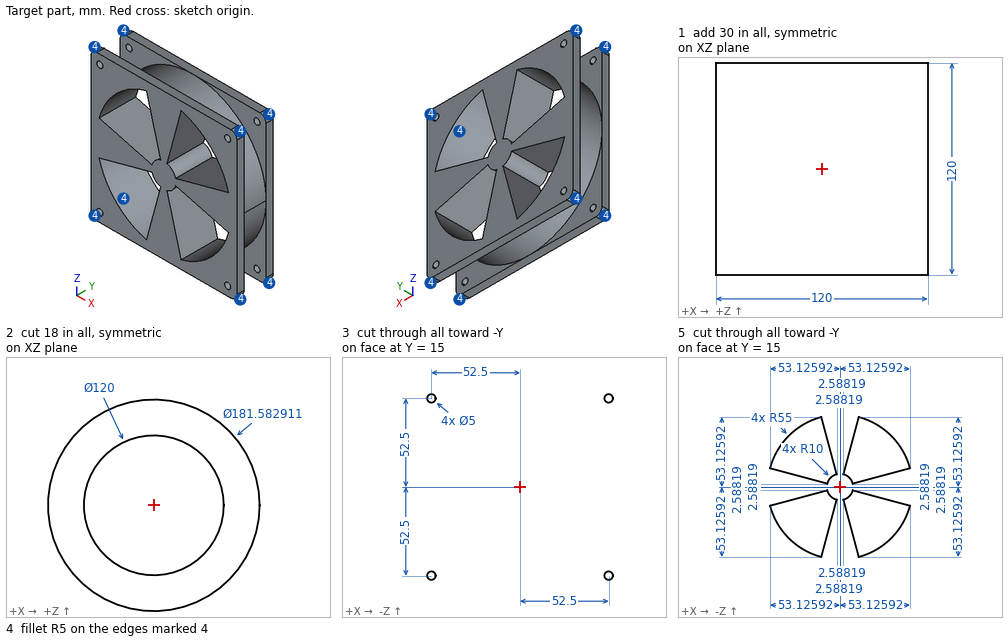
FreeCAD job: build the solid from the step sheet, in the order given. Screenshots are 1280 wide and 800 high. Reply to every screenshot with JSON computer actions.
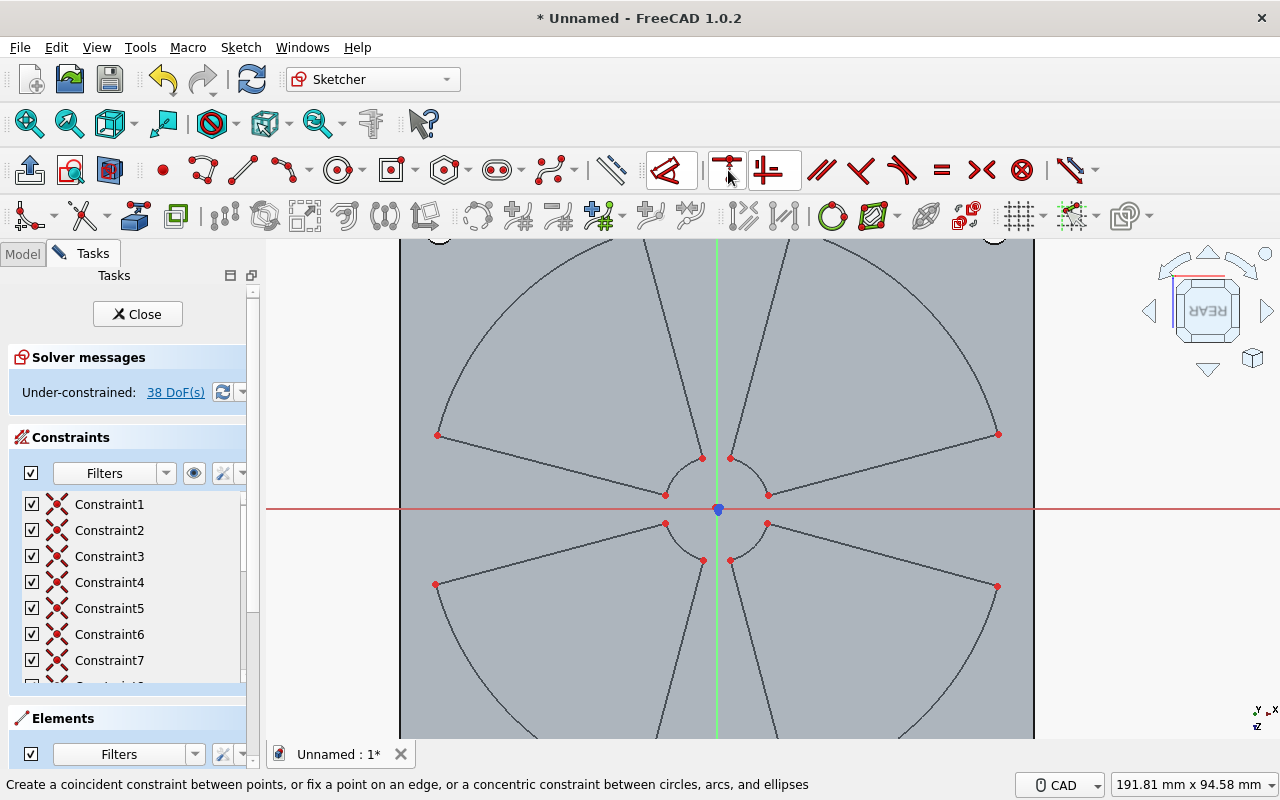
{"action": "left_click", "coordinate": [473, 353]}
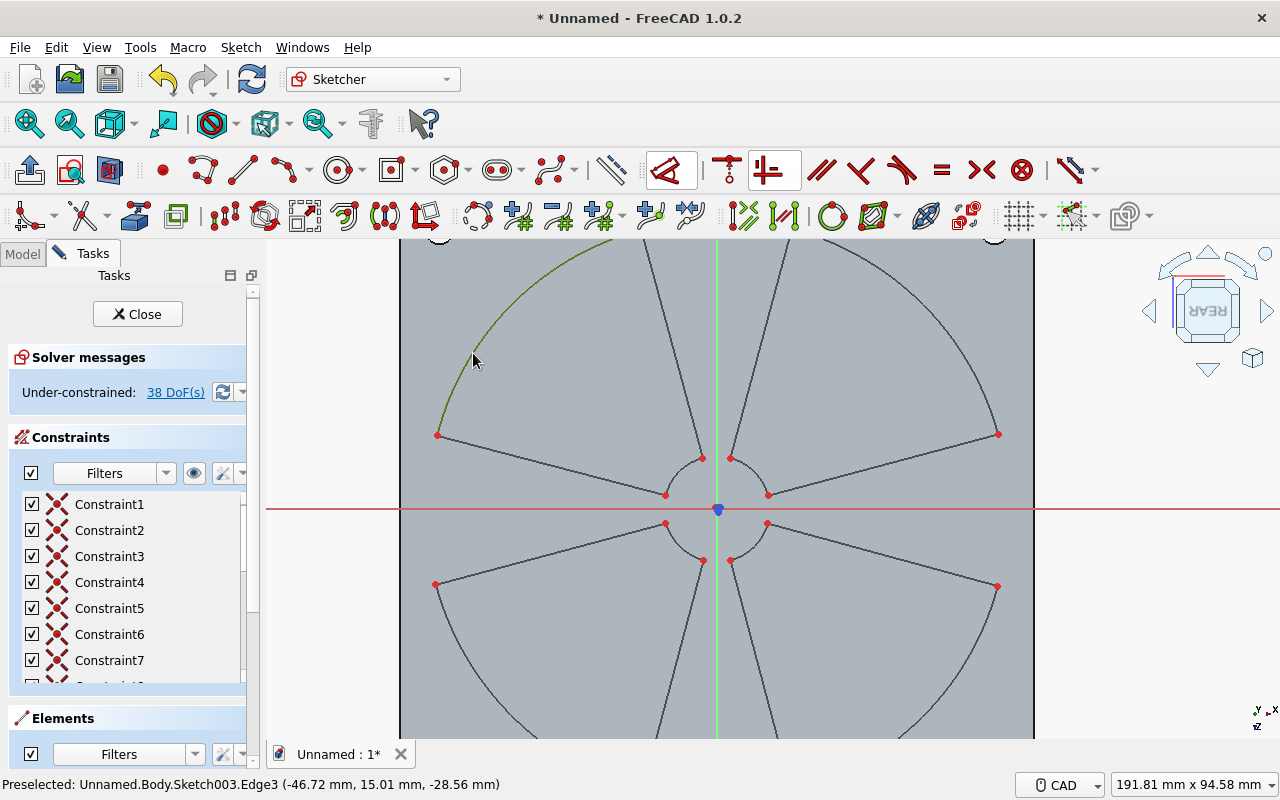
{"action": "left_click", "coordinate": [761, 481]}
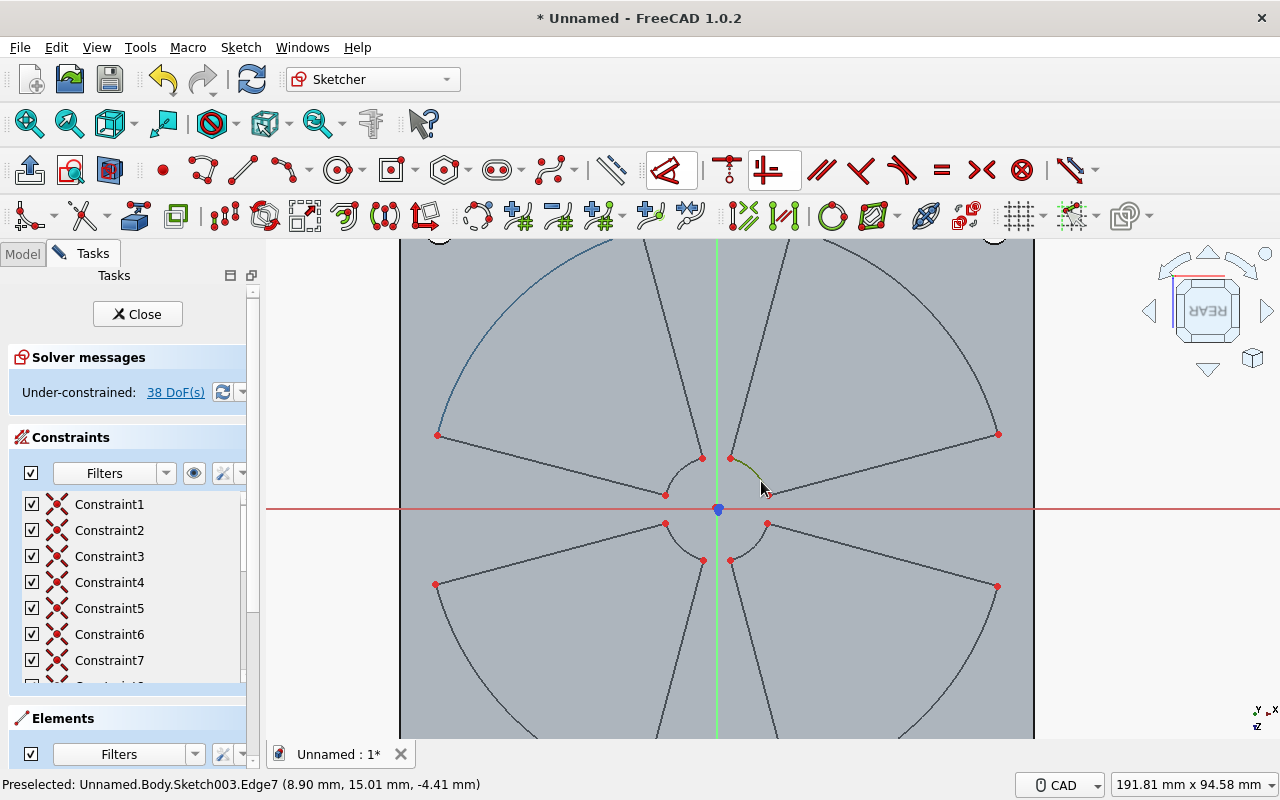
{"action": "left_click", "coordinate": [728, 170]}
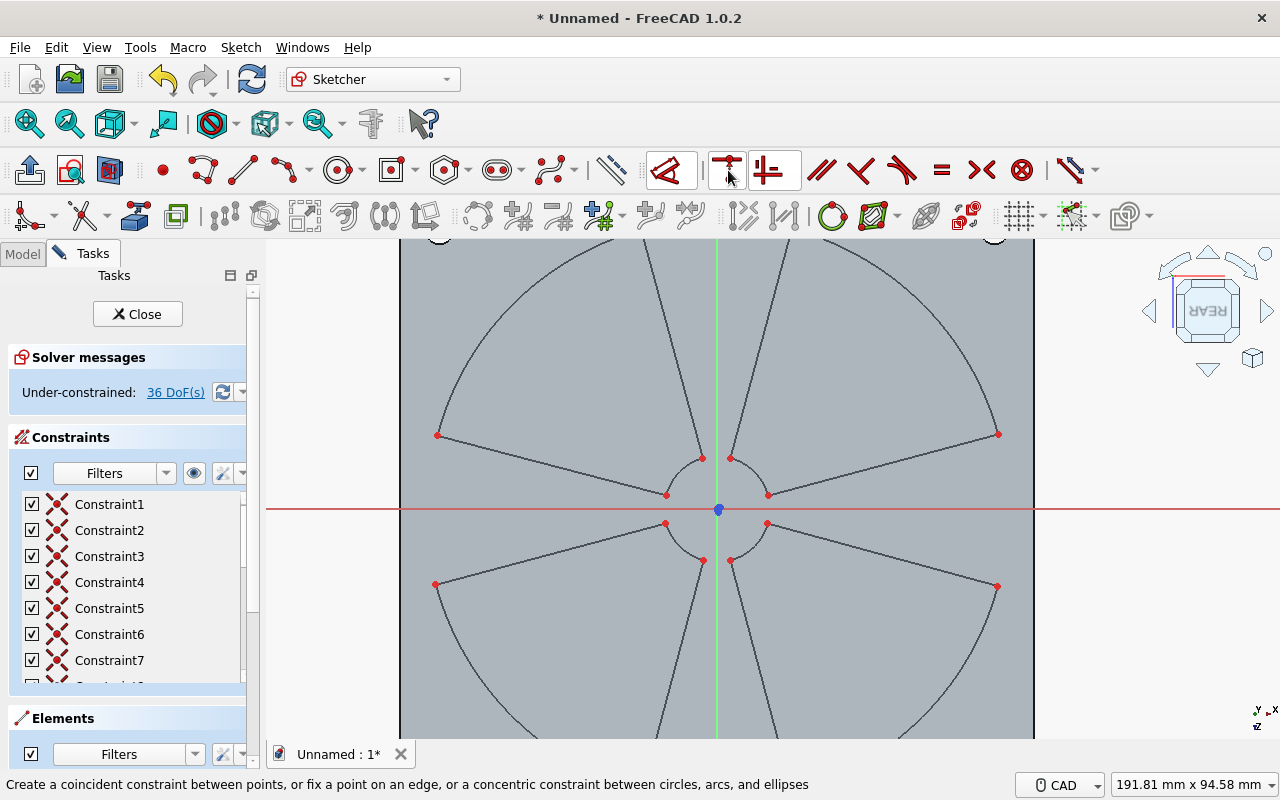
{"action": "left_click", "coordinate": [559, 267]}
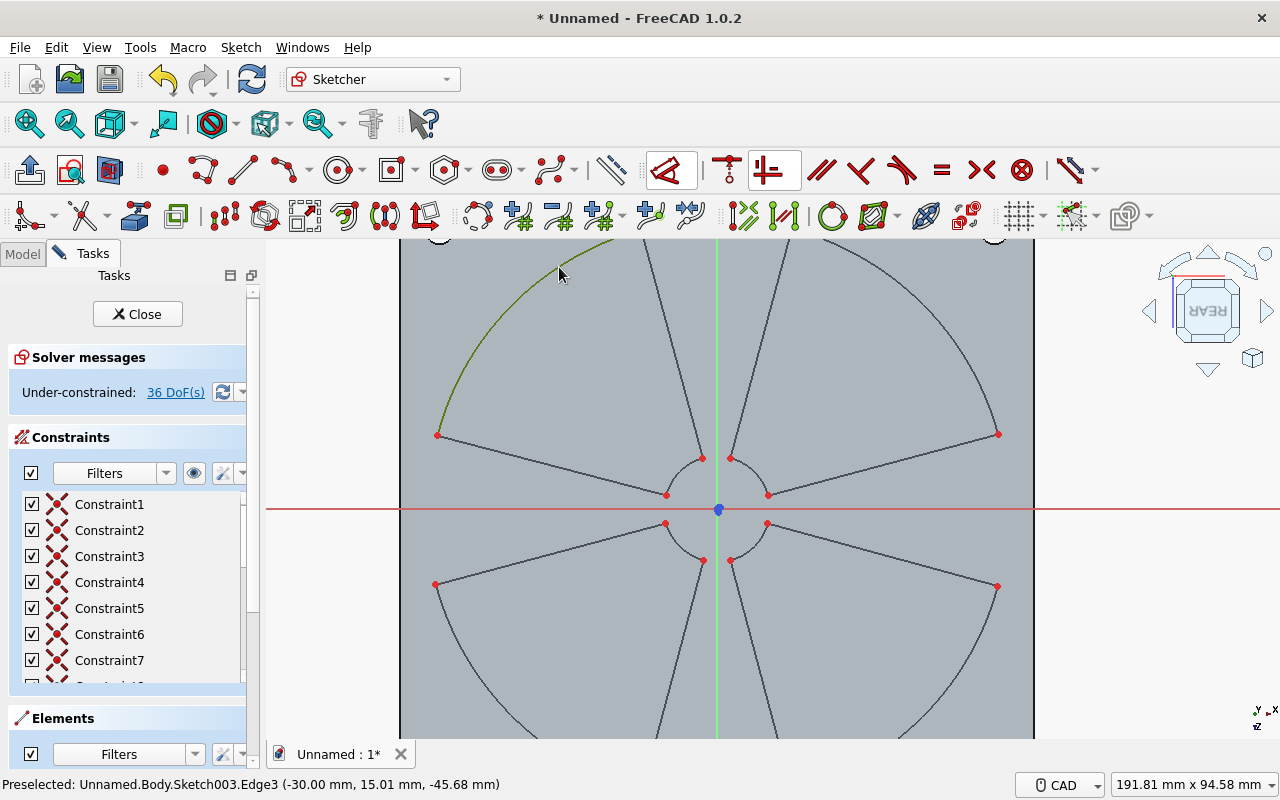
{"action": "left_click", "coordinate": [961, 351]}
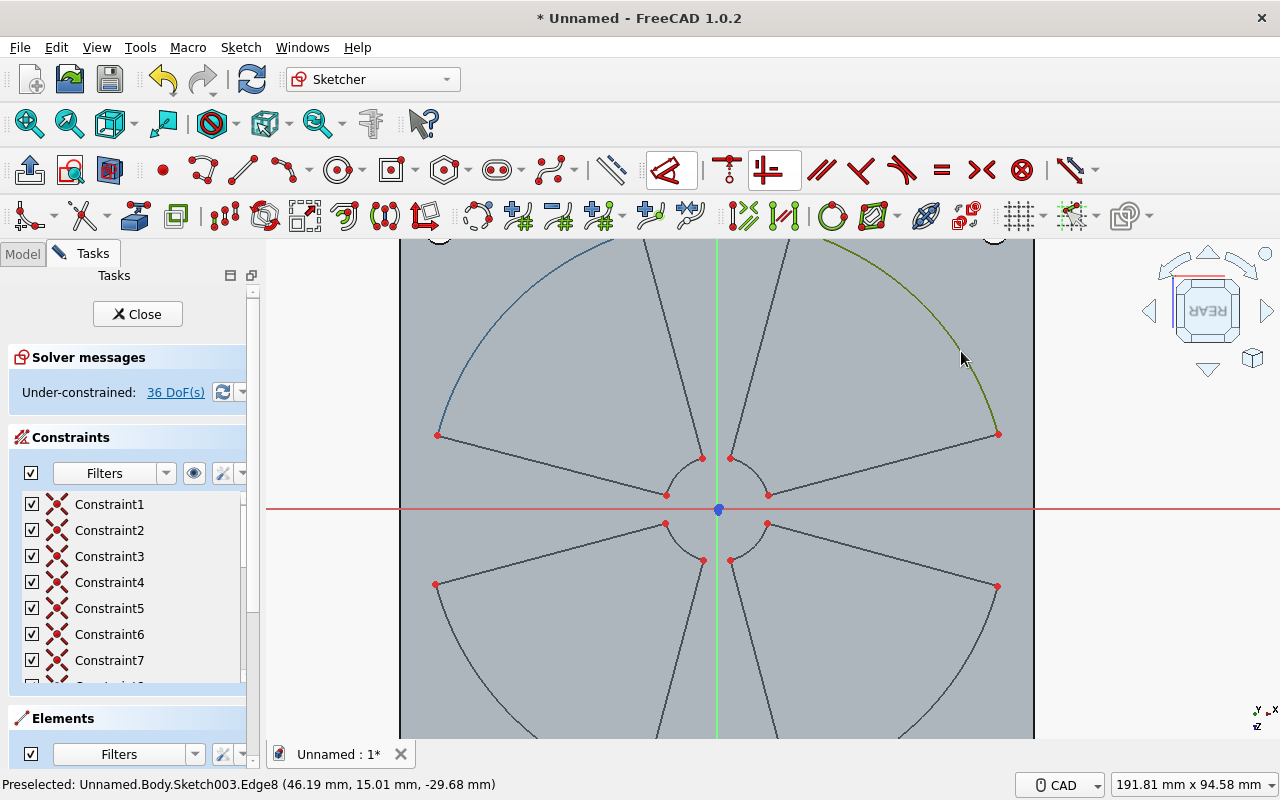
{"action": "left_click", "coordinate": [728, 170]}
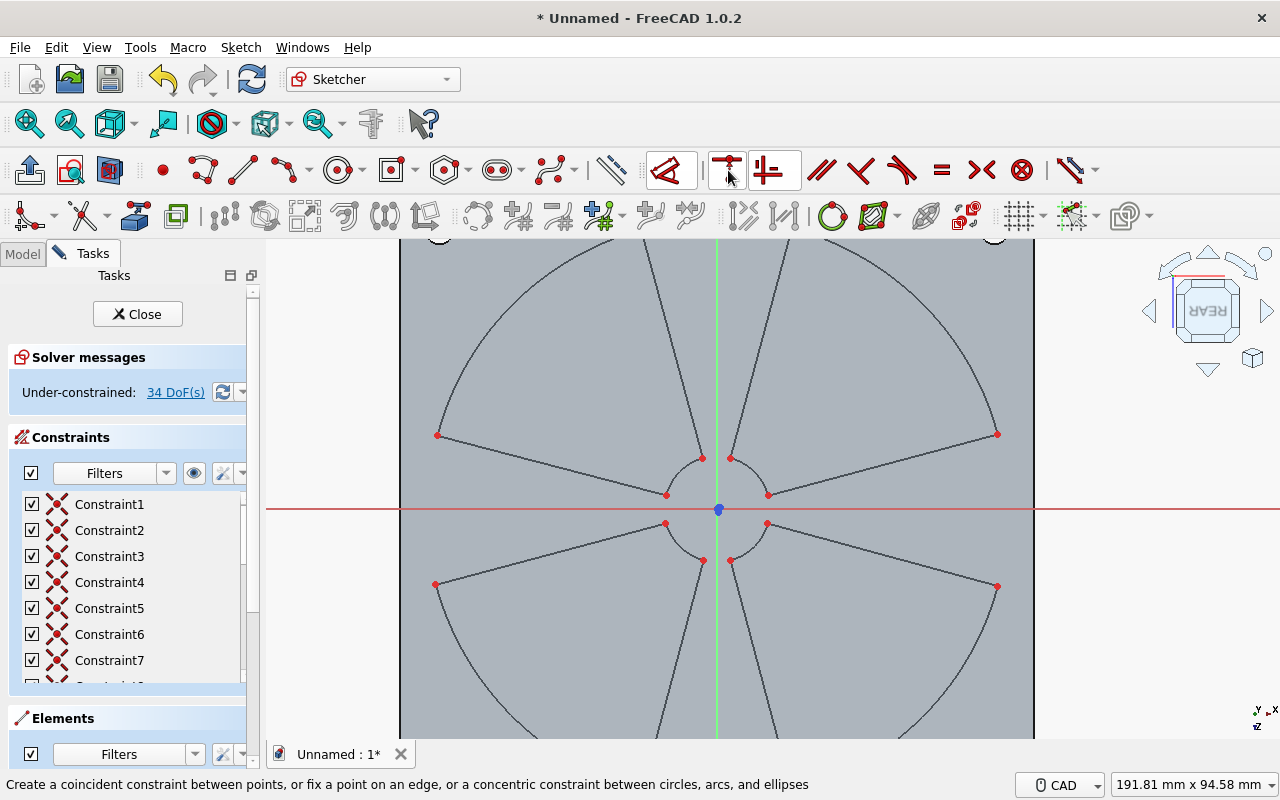
{"action": "left_click", "coordinate": [559, 267]}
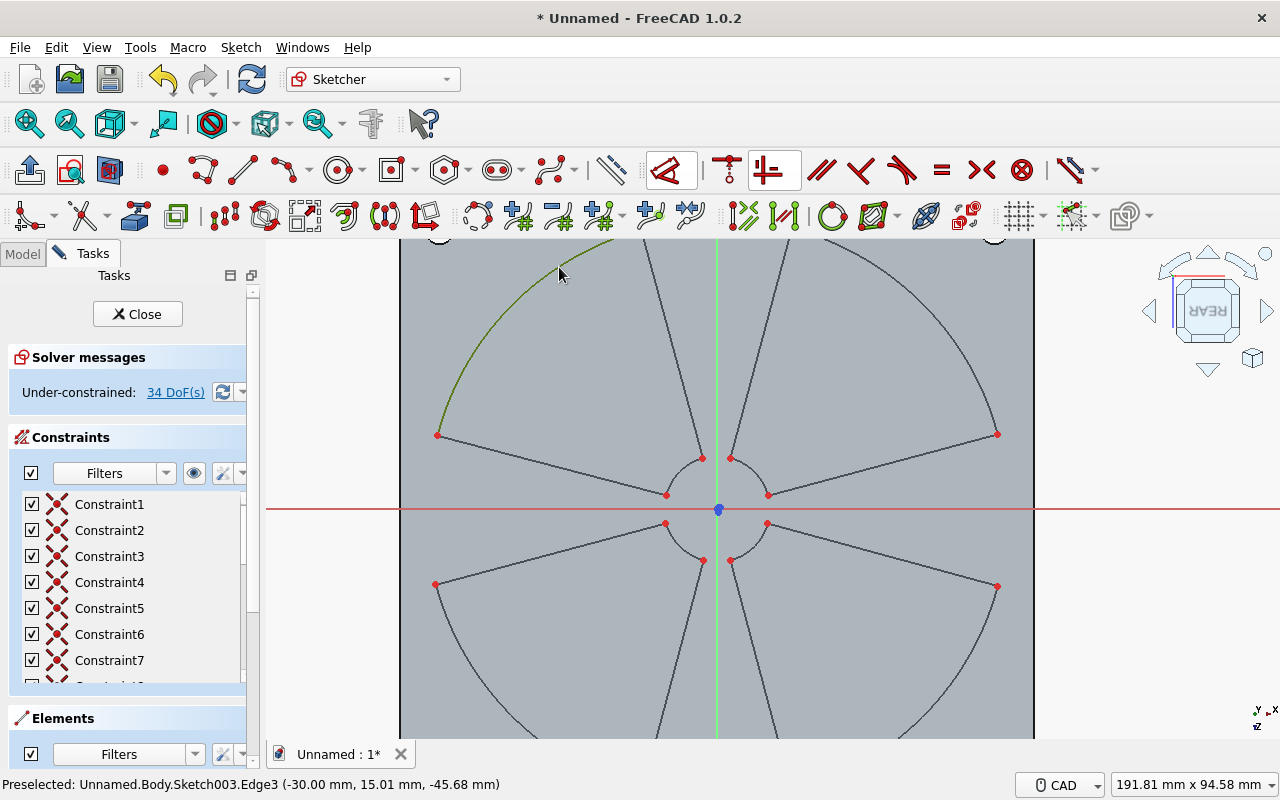
{"action": "left_click", "coordinate": [961, 669]}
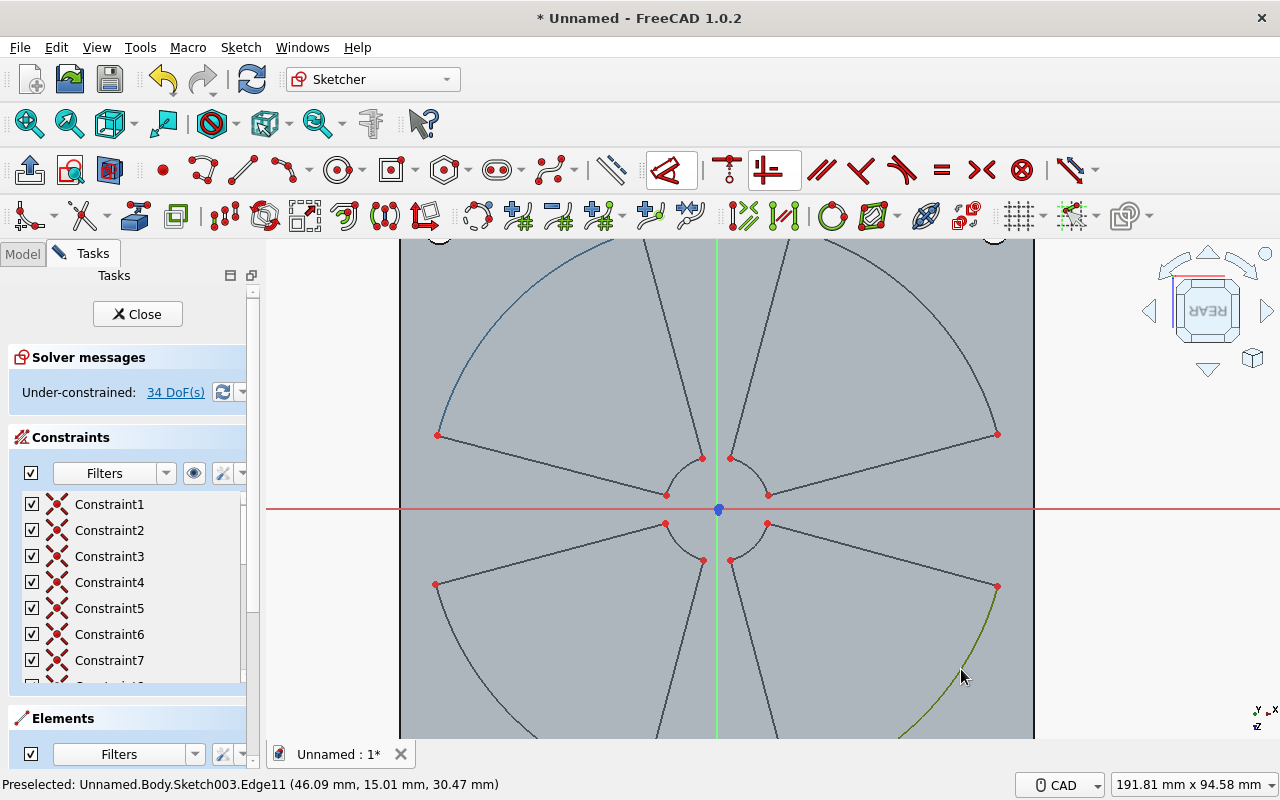
{"action": "left_click", "coordinate": [728, 170]}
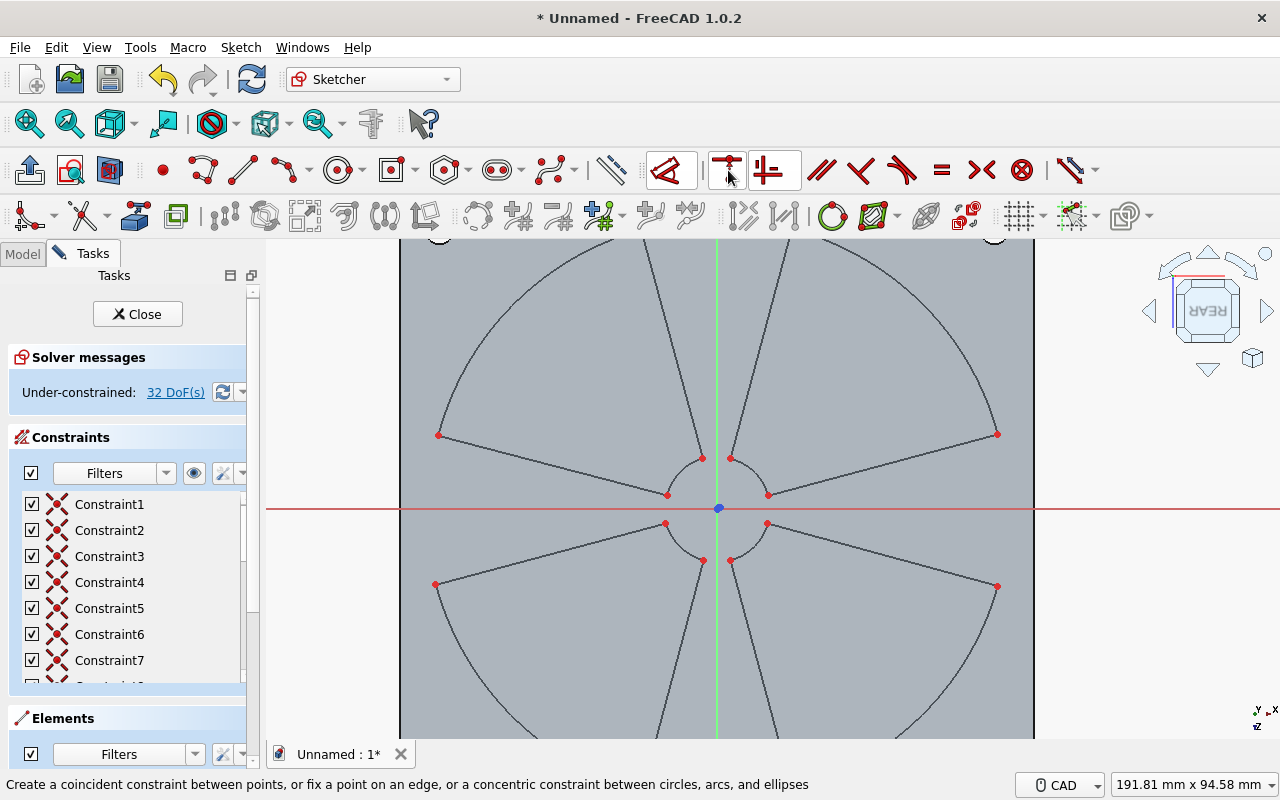
{"action": "left_click", "coordinate": [559, 267]}